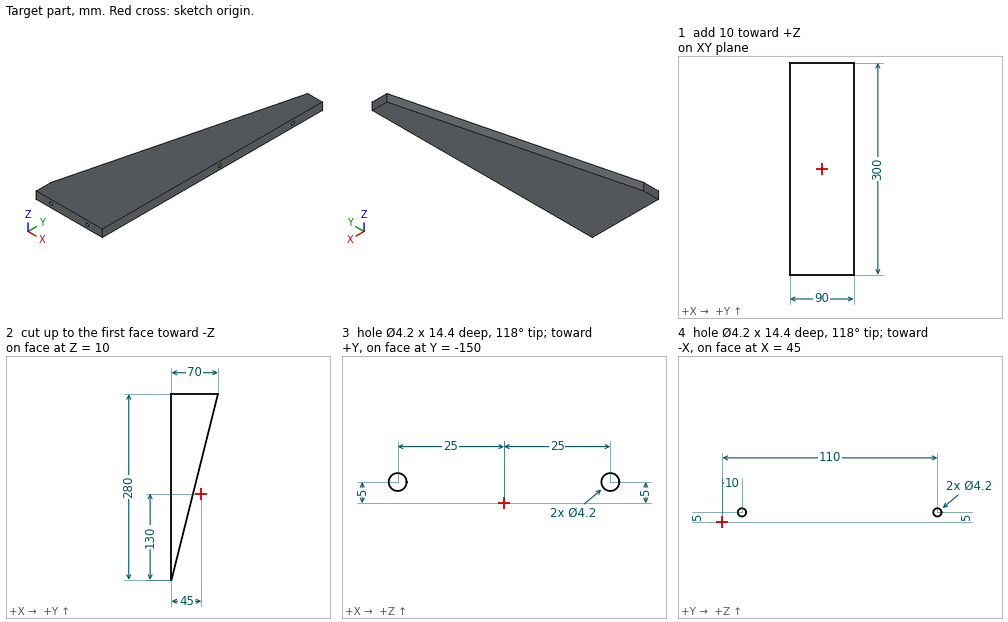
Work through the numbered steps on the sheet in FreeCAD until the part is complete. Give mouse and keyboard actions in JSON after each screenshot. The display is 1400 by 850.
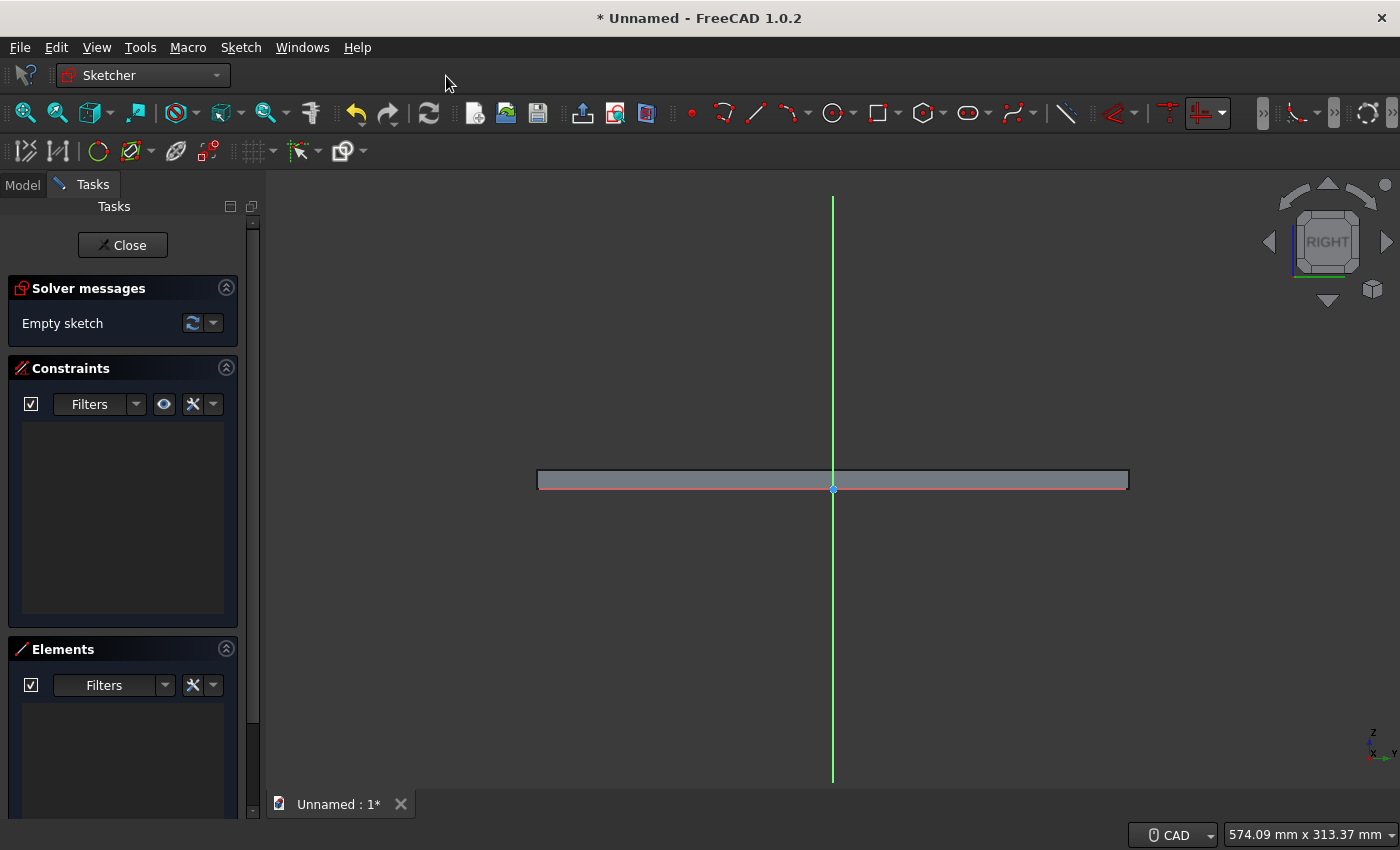
{"action": "scroll", "coordinate": [1048, 484], "scroll_direction": "up", "scroll_amount": 5}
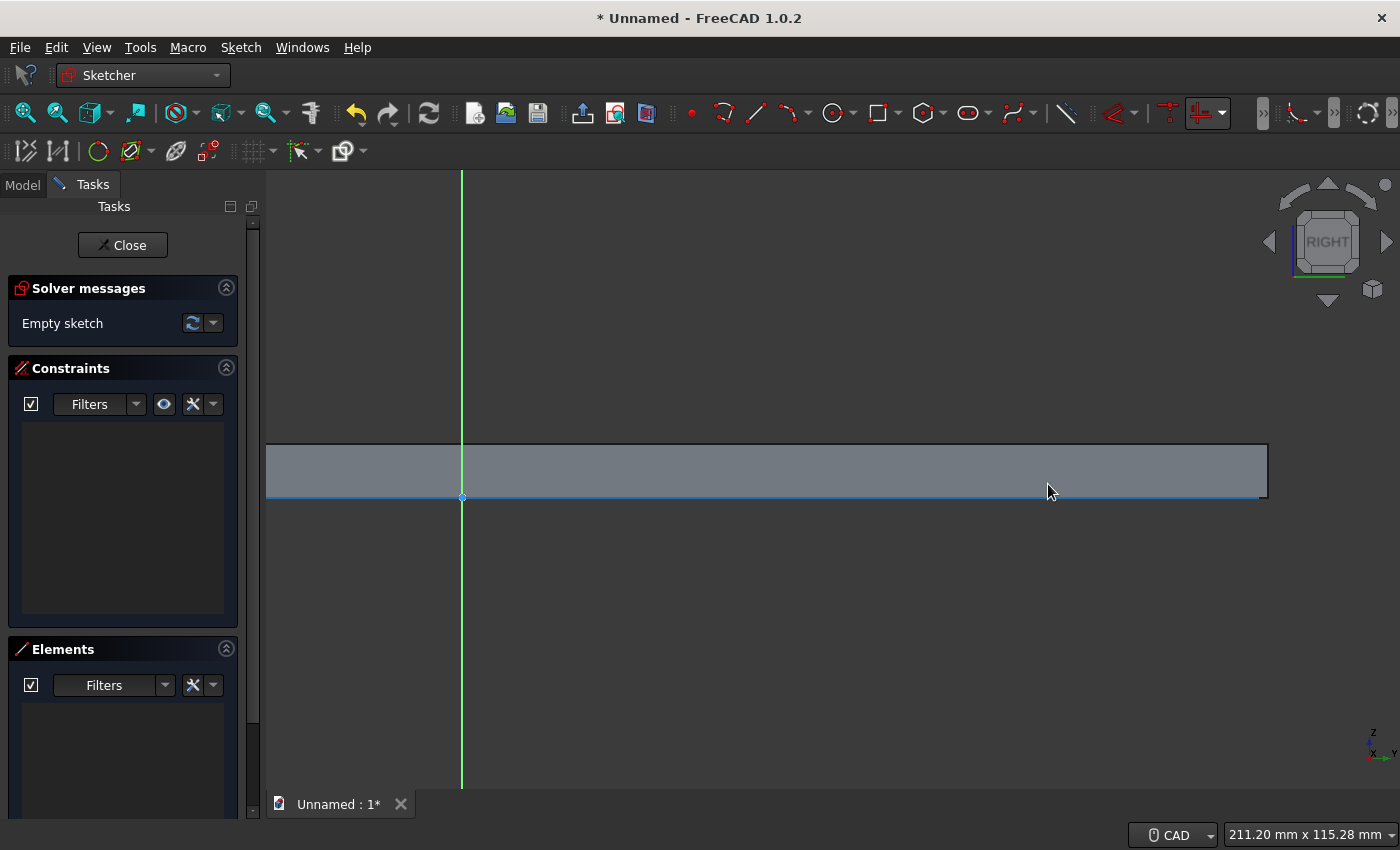
{"action": "key", "text": "g c"}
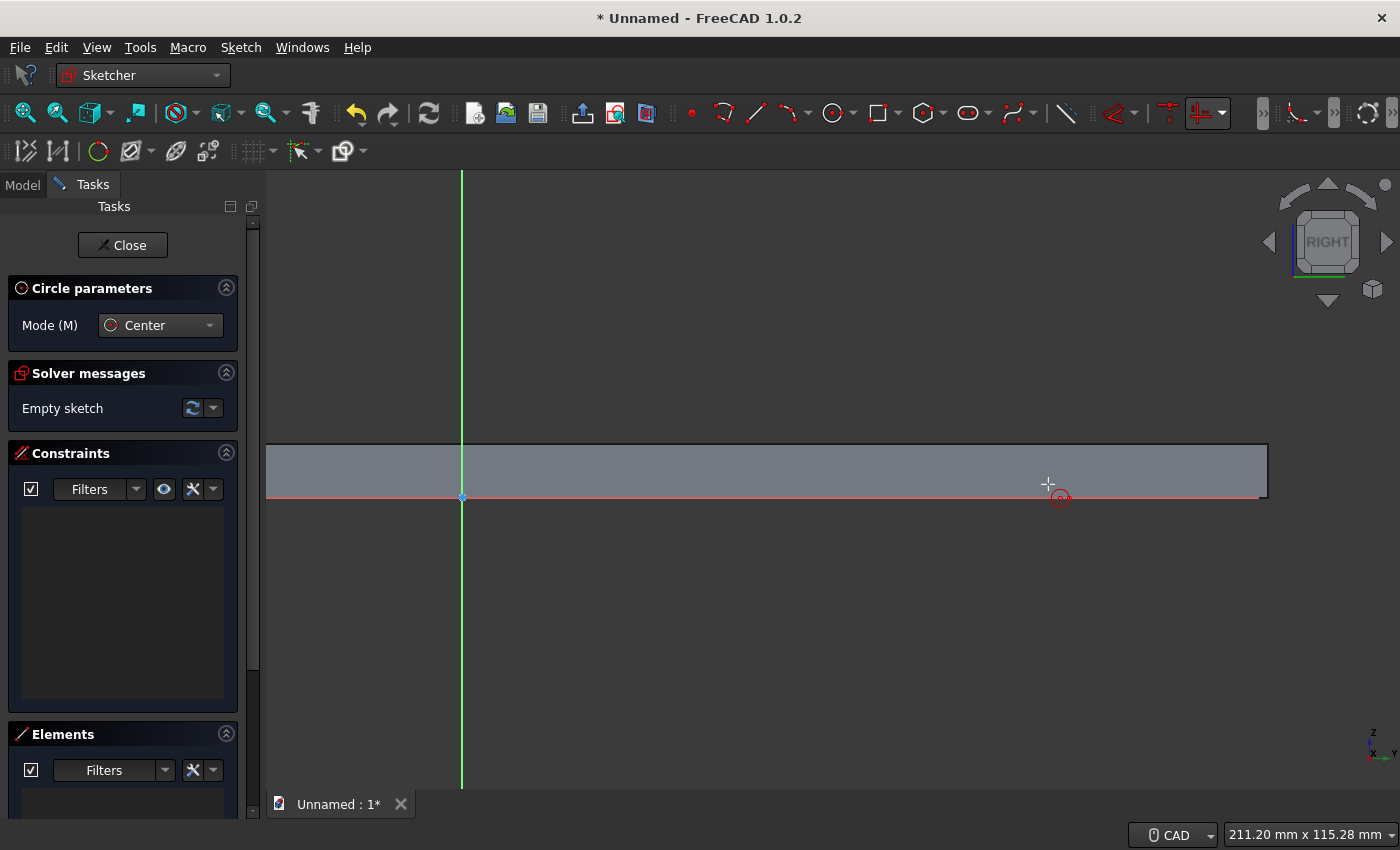
{"action": "scroll", "coordinate": [1053, 471], "scroll_direction": "up", "scroll_amount": 4}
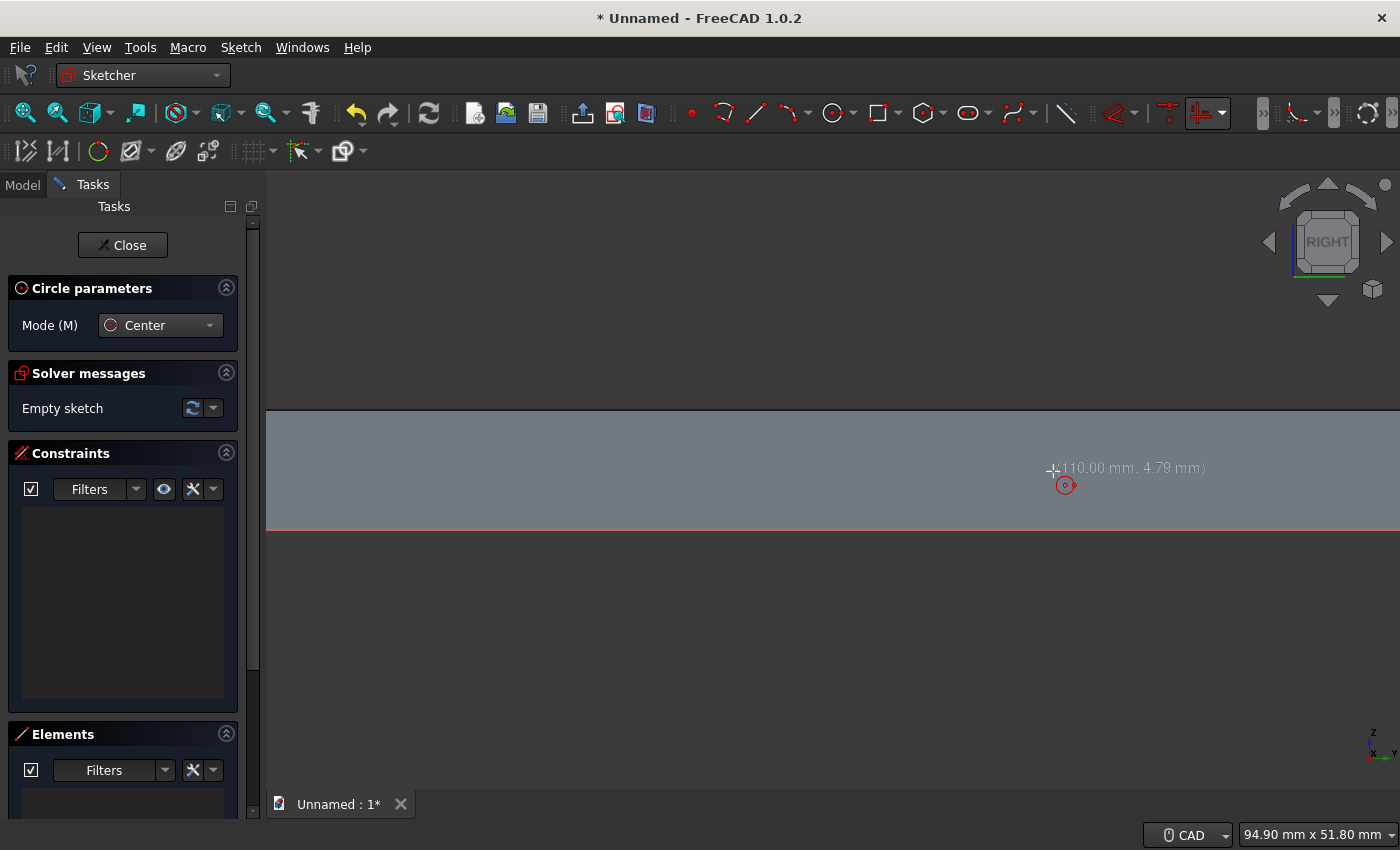
{"action": "left_click", "coordinate": [1052, 470]}
{"action": "left_click", "coordinate": [1070, 452]}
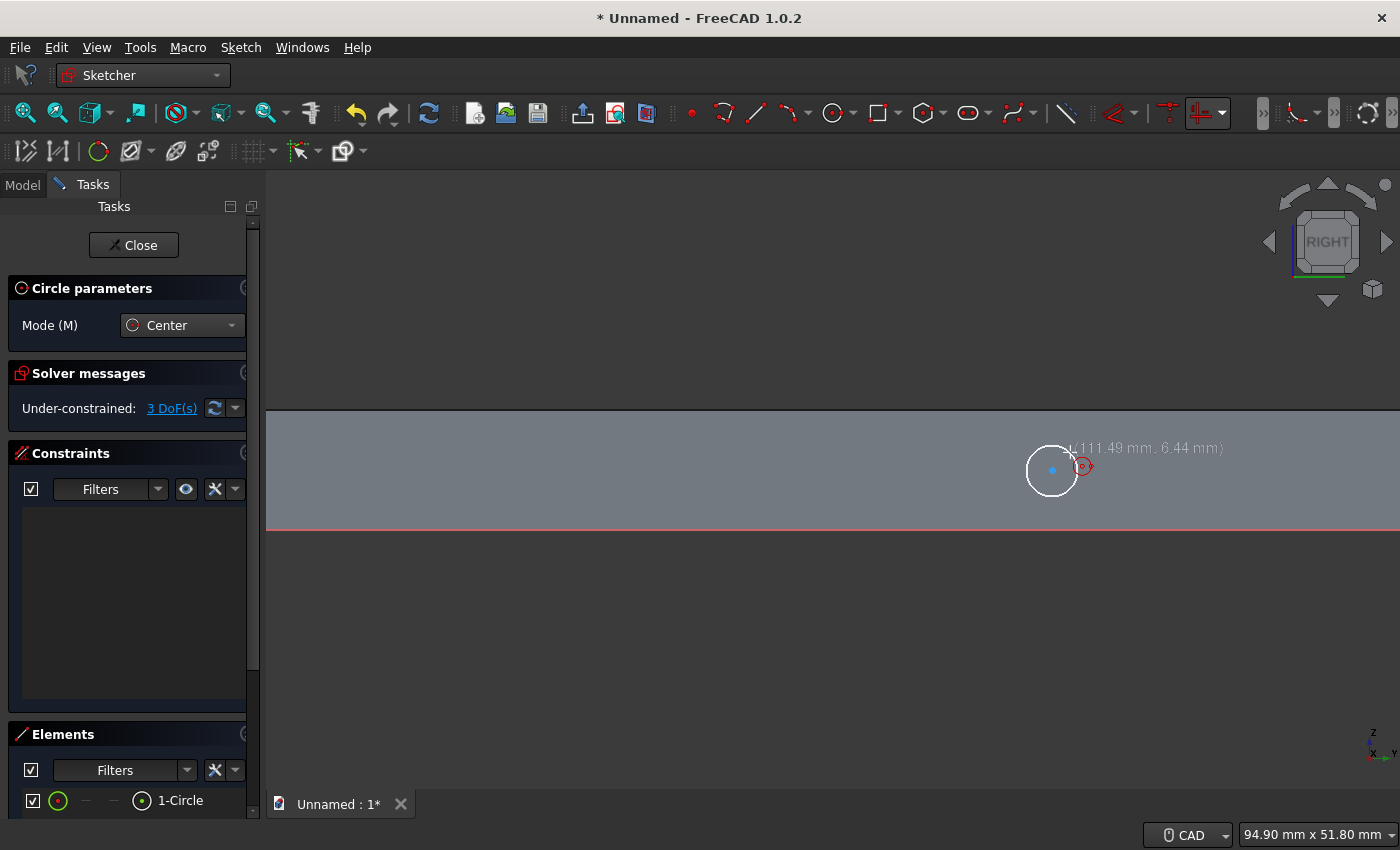
{"action": "scroll", "coordinate": [1056, 473], "scroll_direction": "down", "scroll_amount": 4}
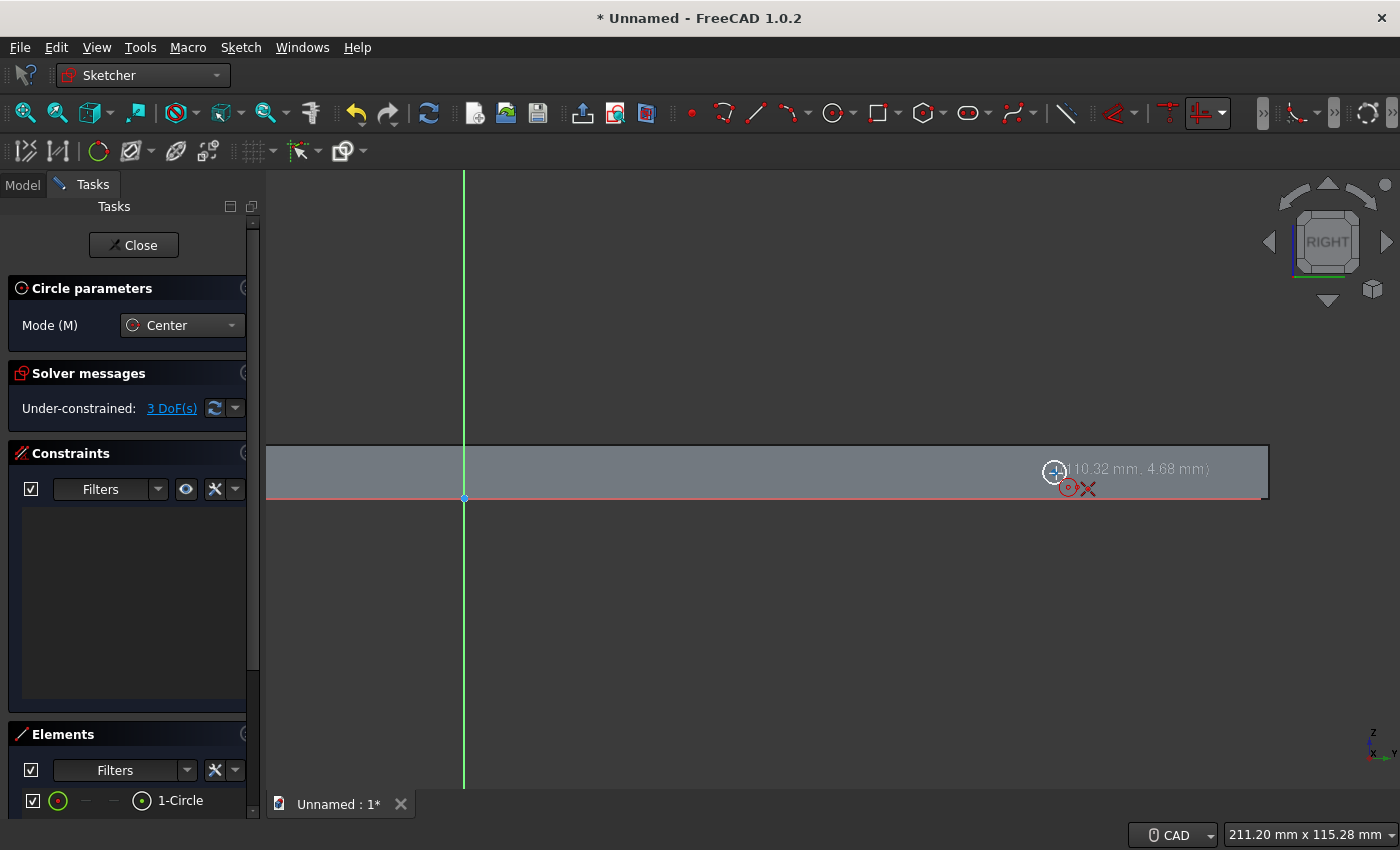
{"action": "scroll", "coordinate": [518, 472], "scroll_direction": "up", "scroll_amount": 4}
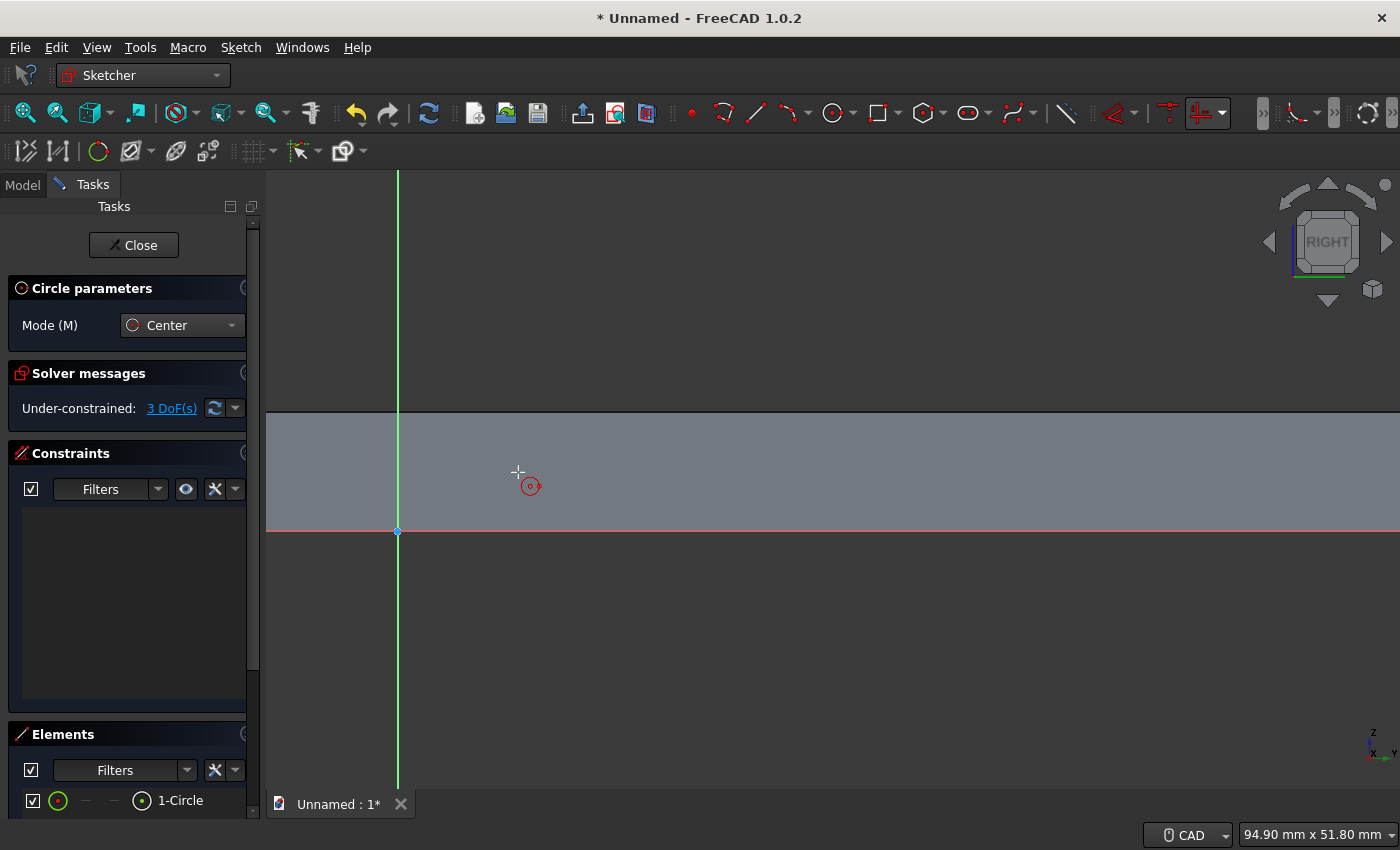
{"action": "left_click", "coordinate": [517, 471]}
{"action": "left_click", "coordinate": [535, 454]}
{"action": "key", "text": "Escape"}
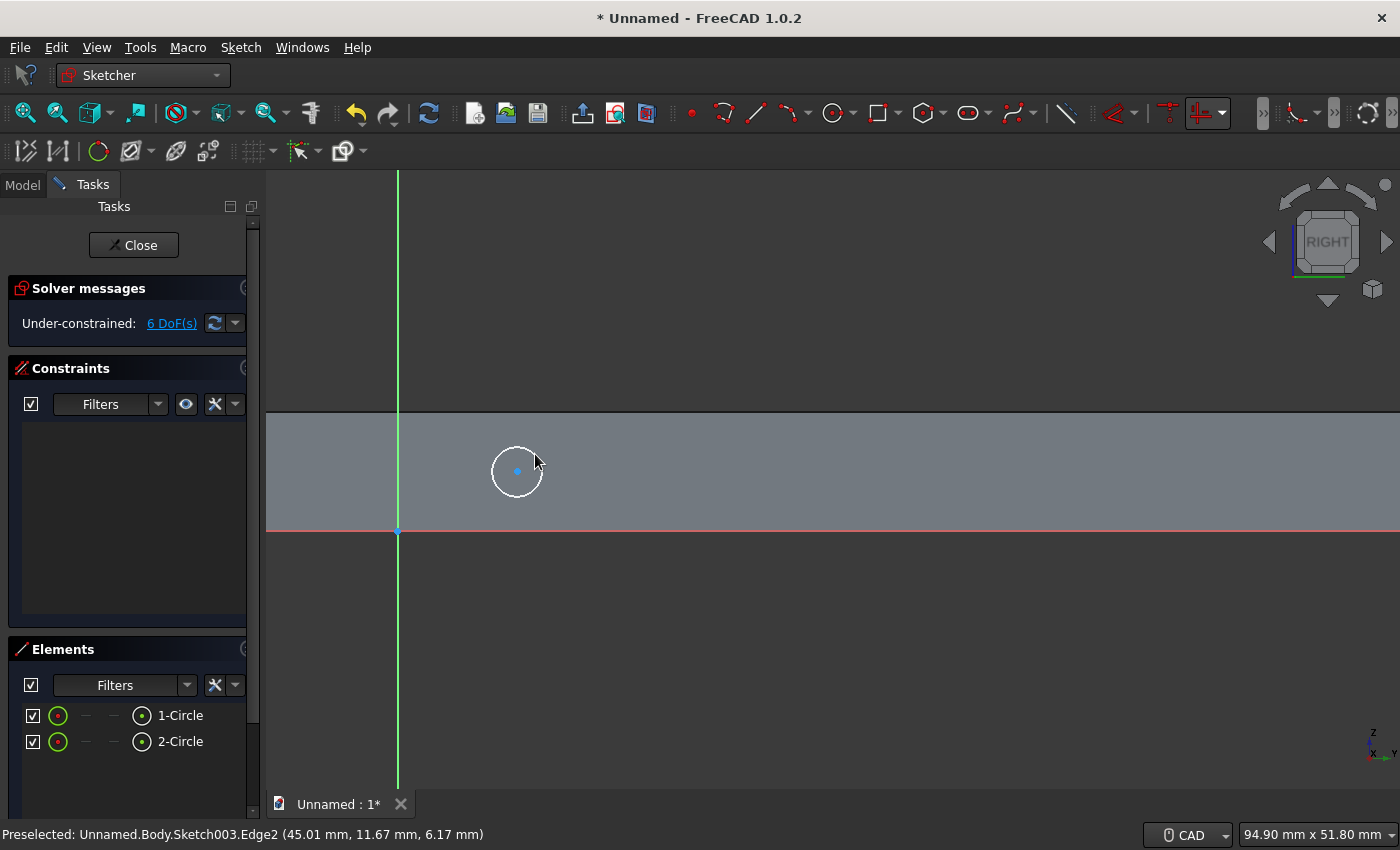
{"action": "scroll", "coordinate": [517, 472], "scroll_direction": "down", "scroll_amount": 4}